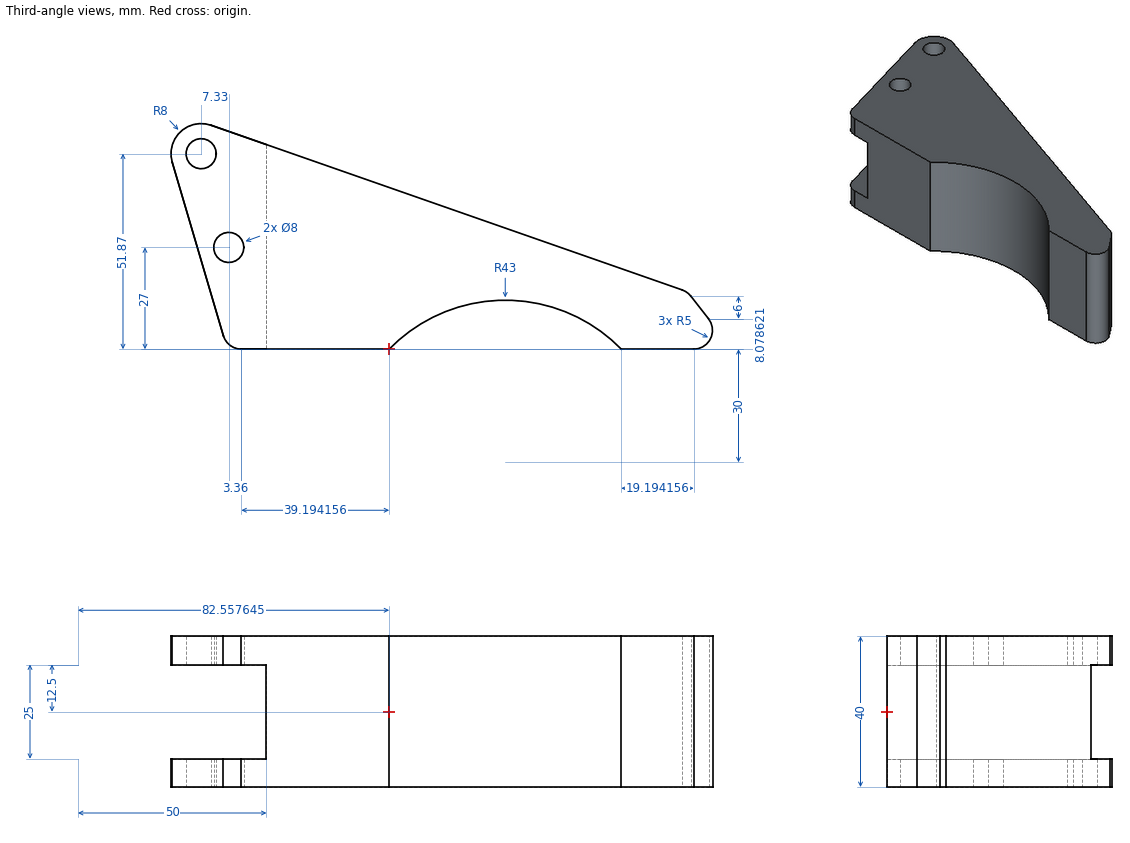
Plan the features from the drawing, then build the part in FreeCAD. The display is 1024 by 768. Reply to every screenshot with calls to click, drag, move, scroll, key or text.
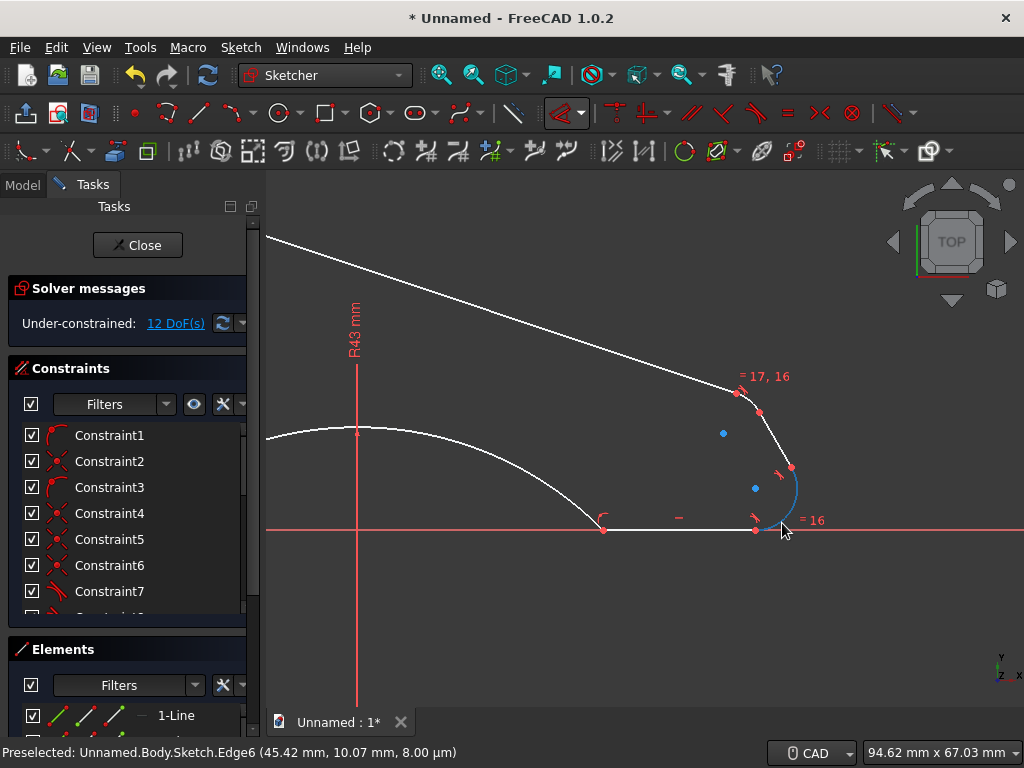
click(780, 522)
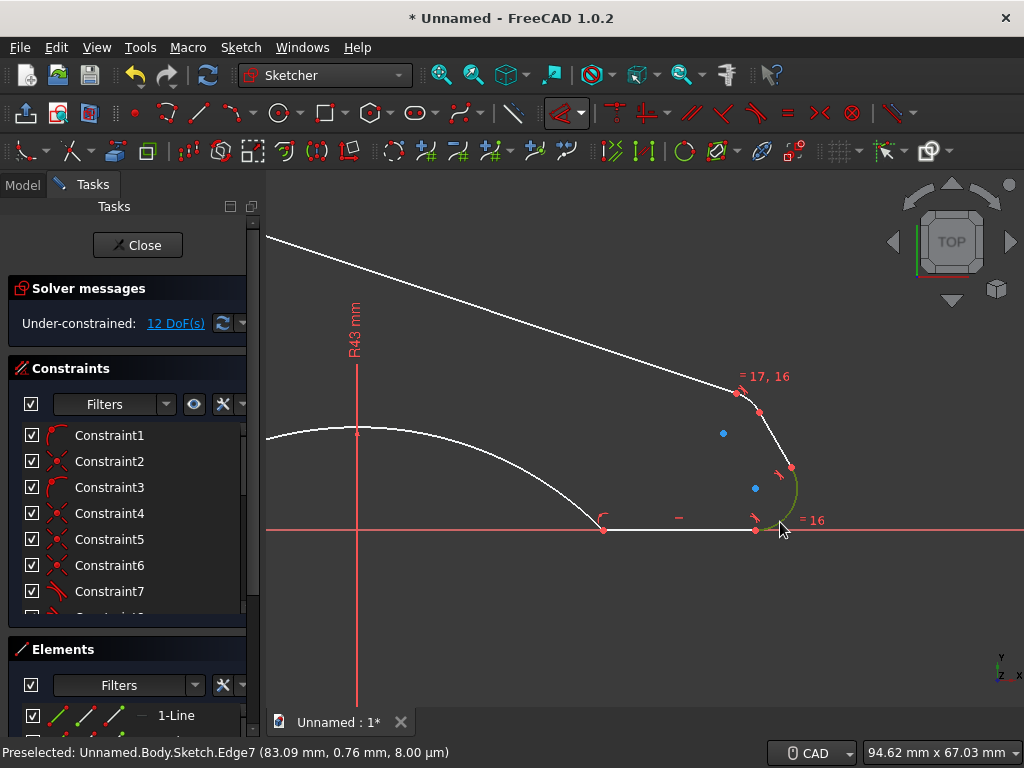
click(584, 114)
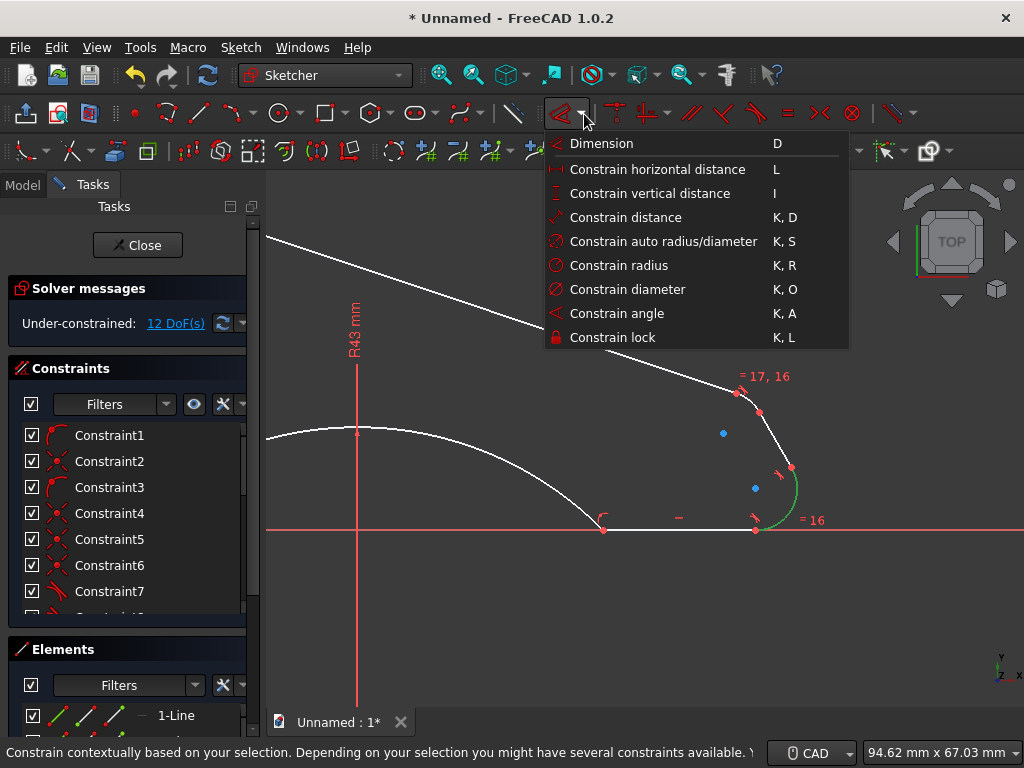
click(697, 265)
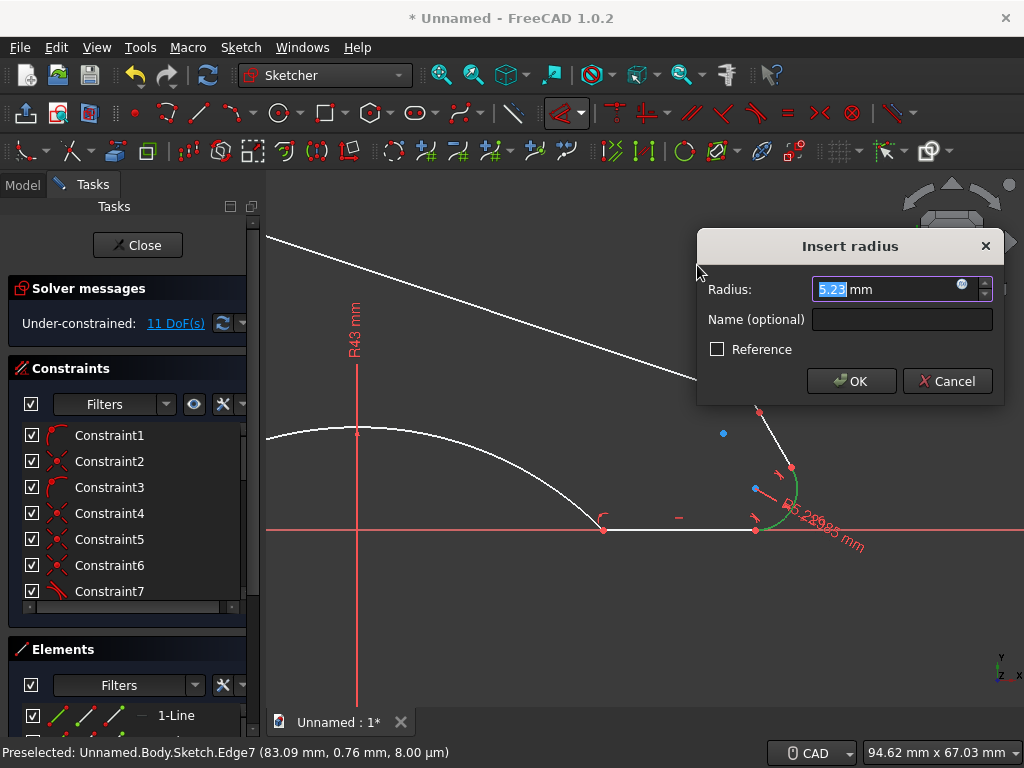
text(5)
key(Return)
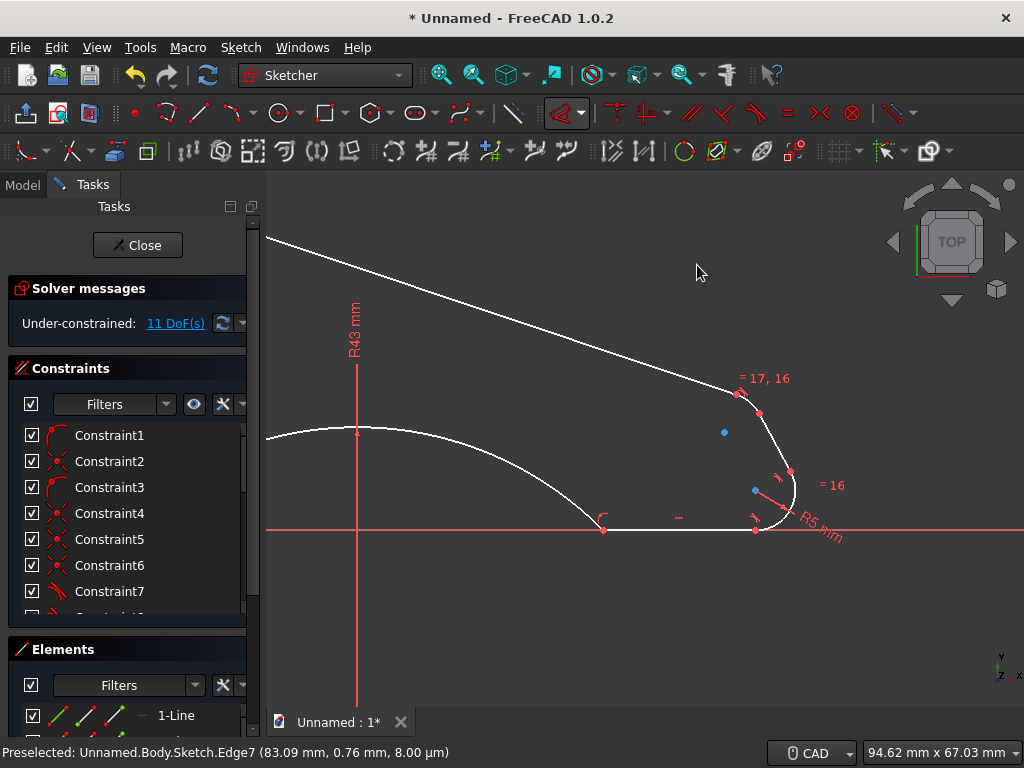
scroll(783, 523, down, 5)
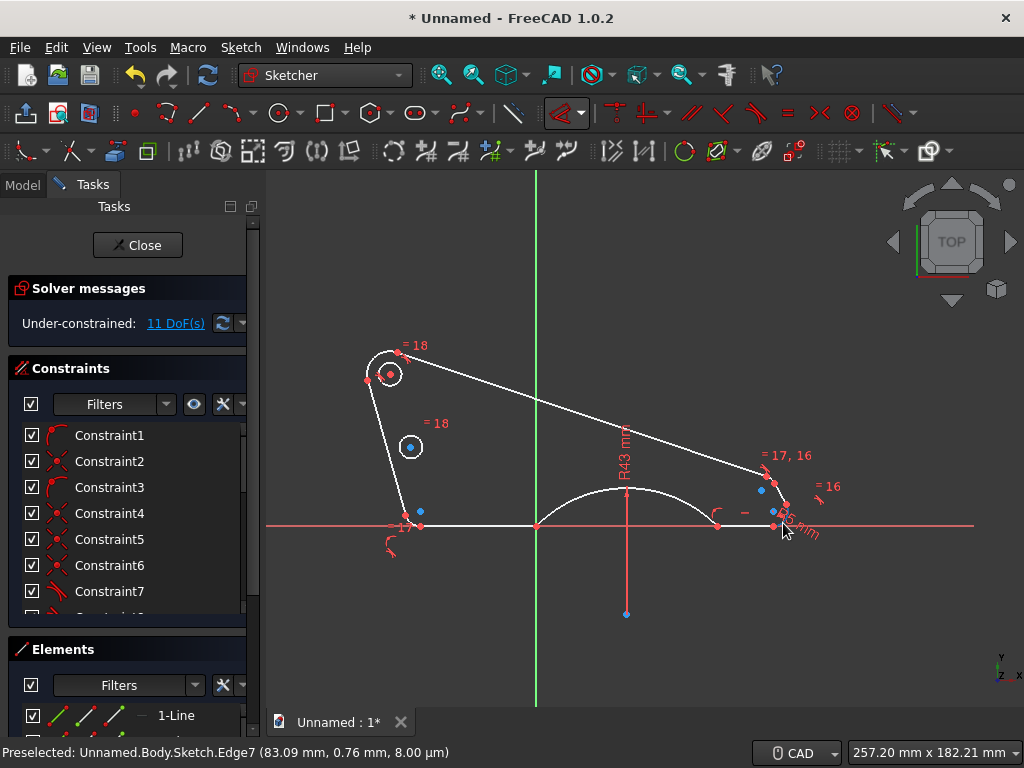
scroll(383, 353, up, 3)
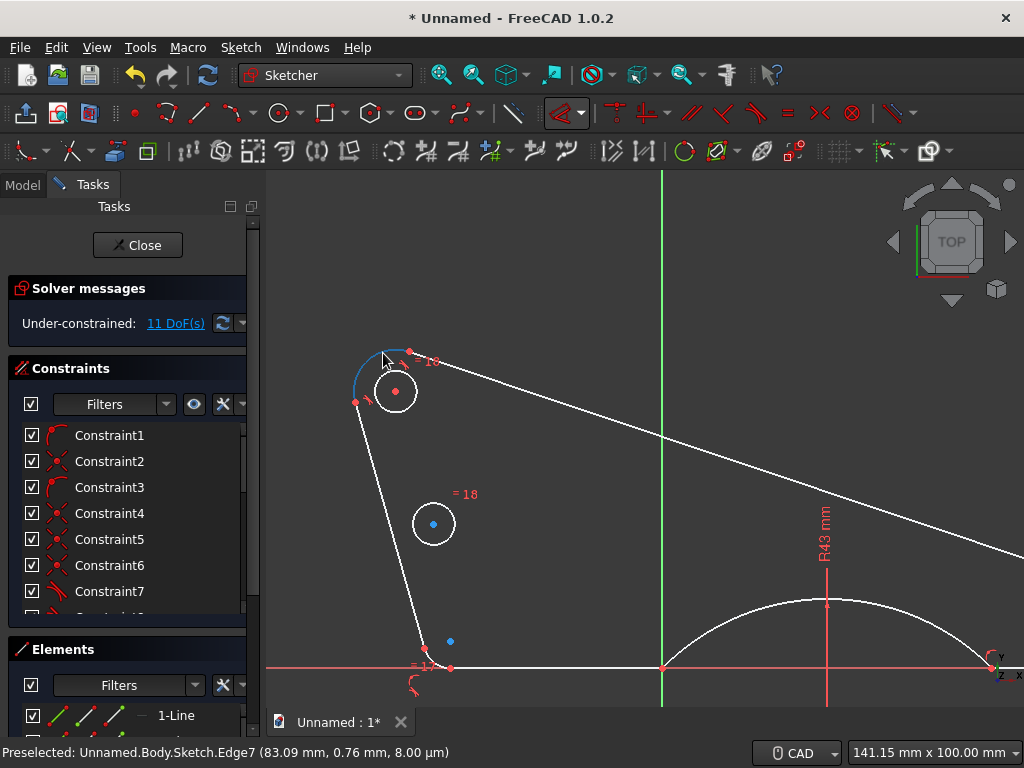
click(382, 352)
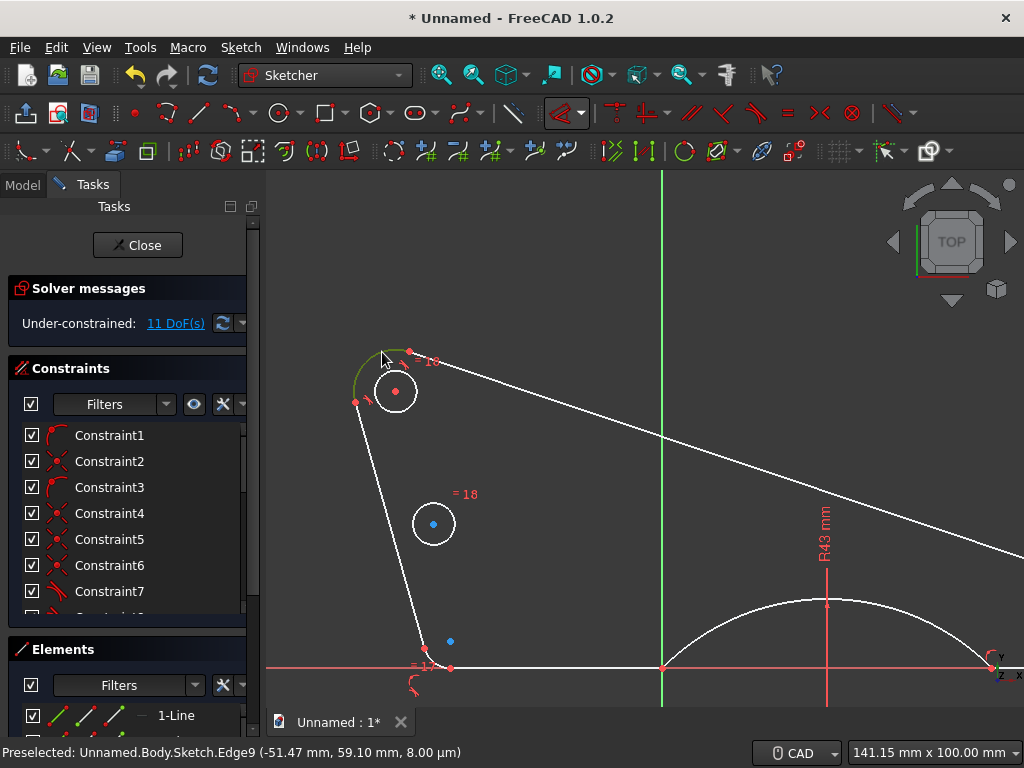
key(k)
key(r)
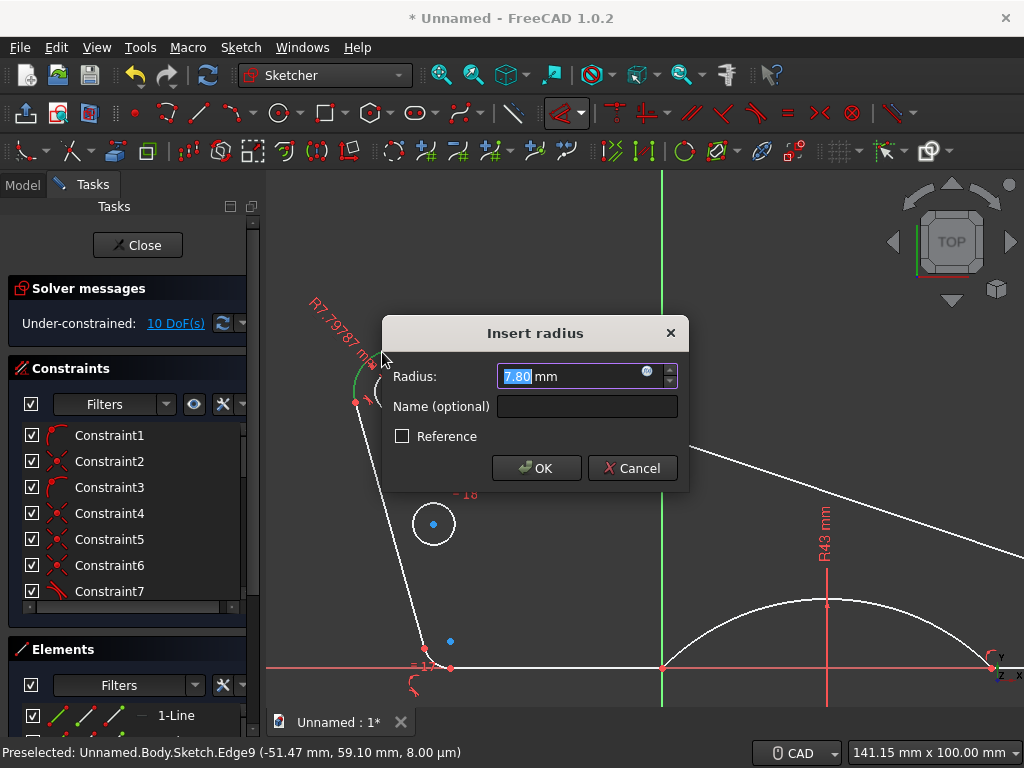
text(8)
key(Return)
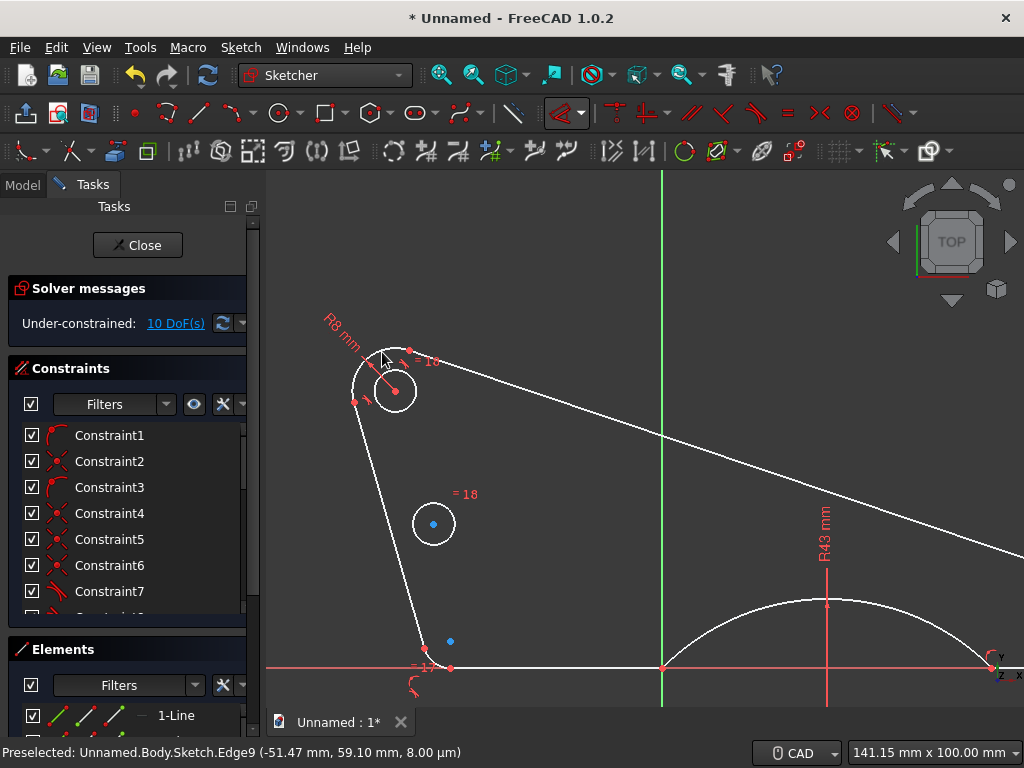
click(449, 509)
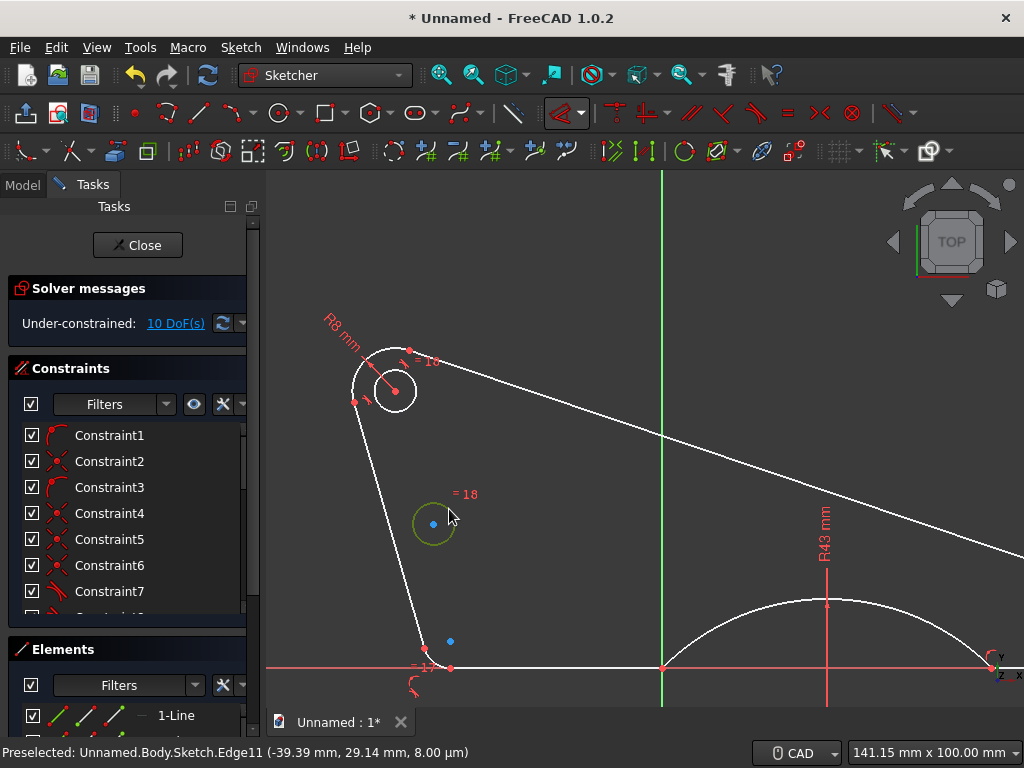
click(584, 114)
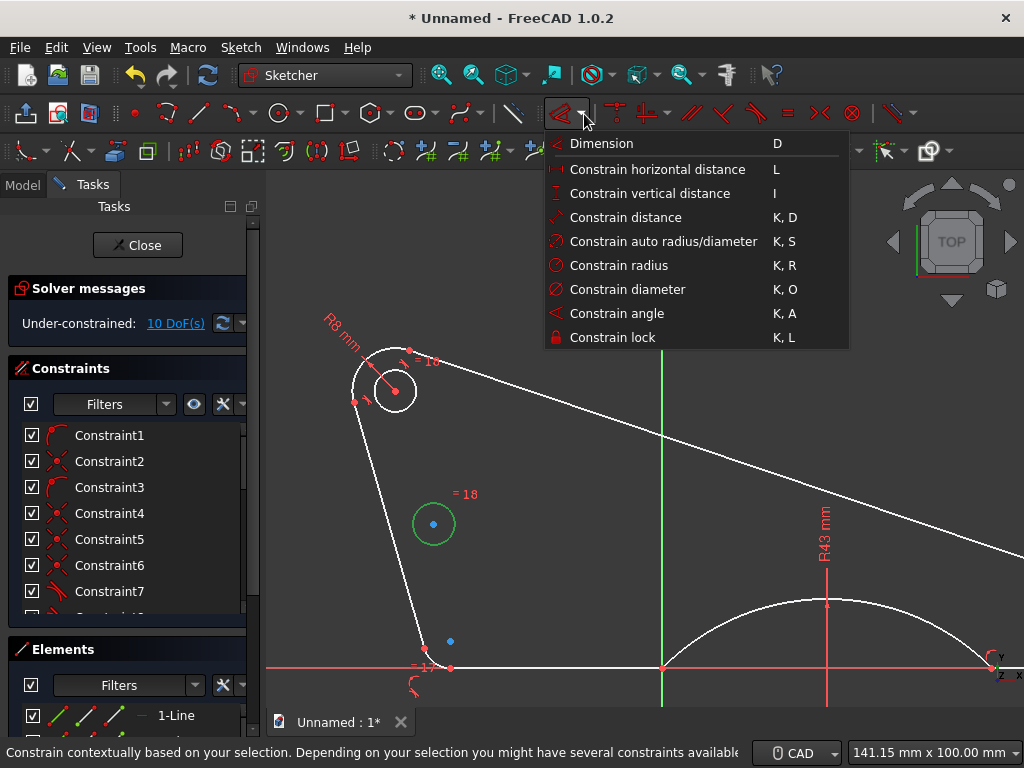
click(697, 289)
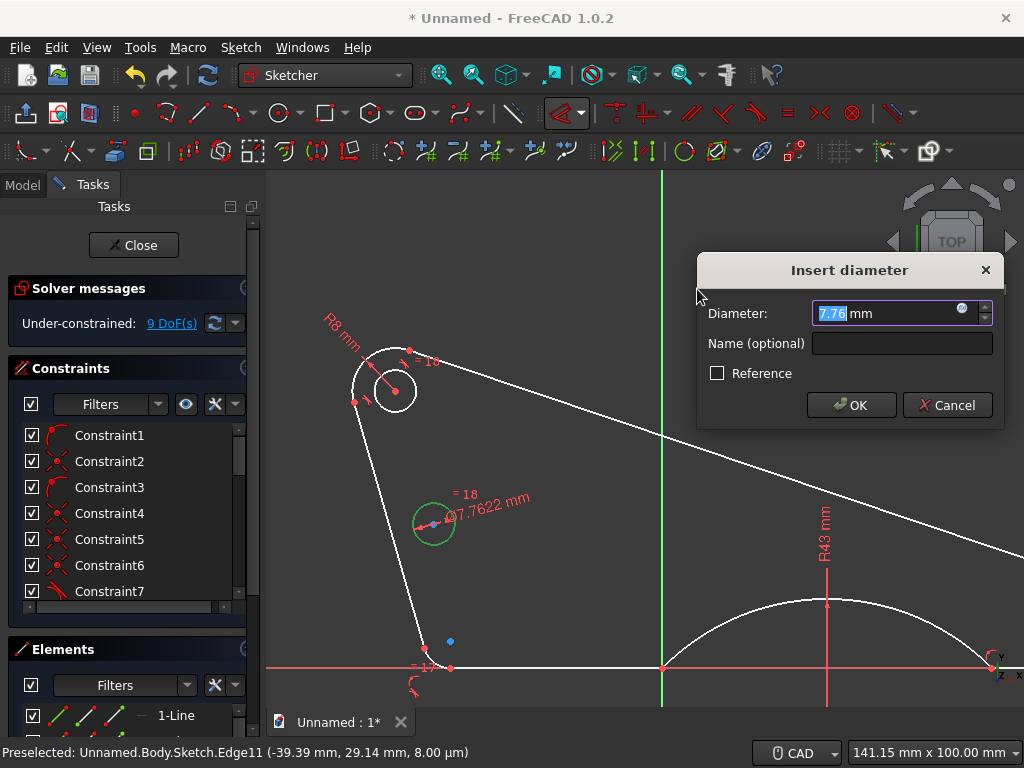
text(8)
key(Return)